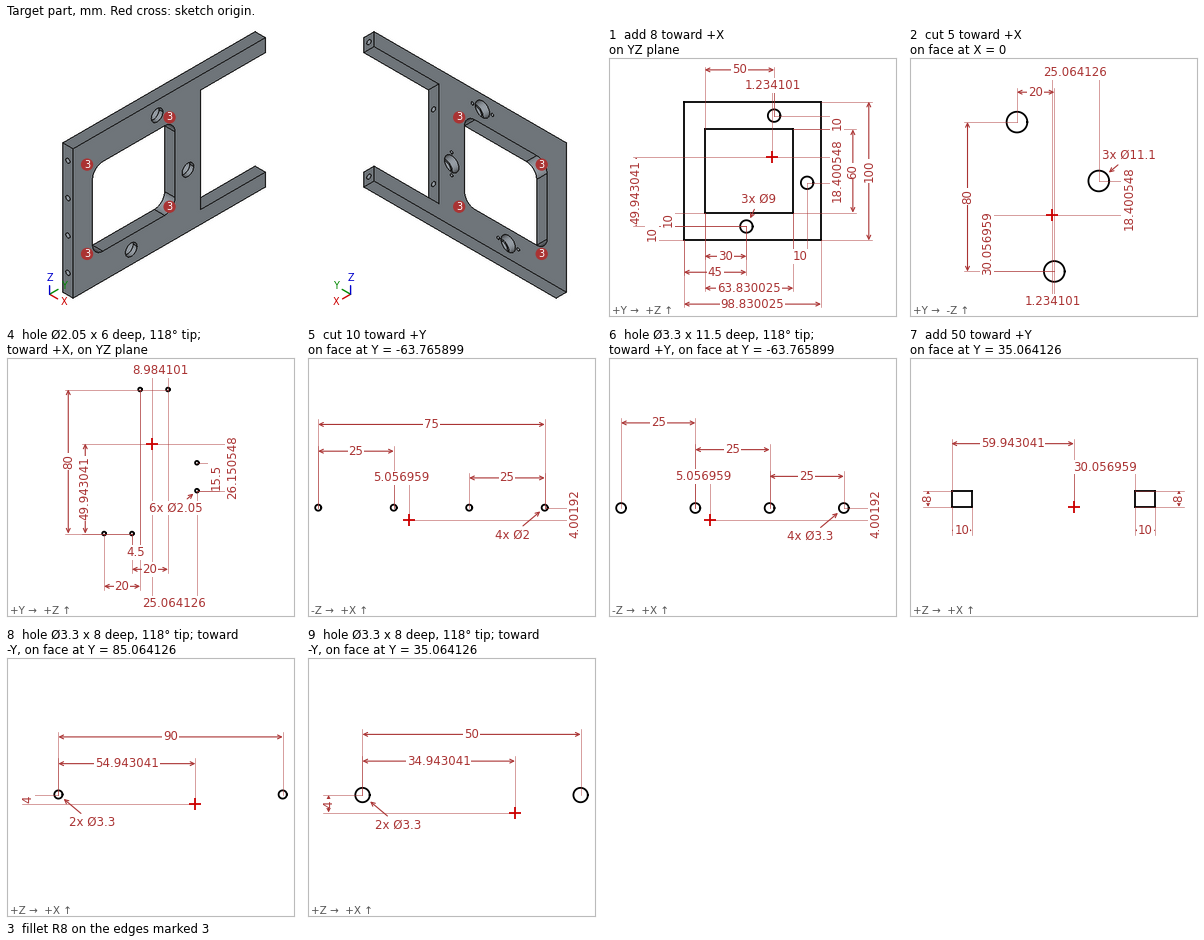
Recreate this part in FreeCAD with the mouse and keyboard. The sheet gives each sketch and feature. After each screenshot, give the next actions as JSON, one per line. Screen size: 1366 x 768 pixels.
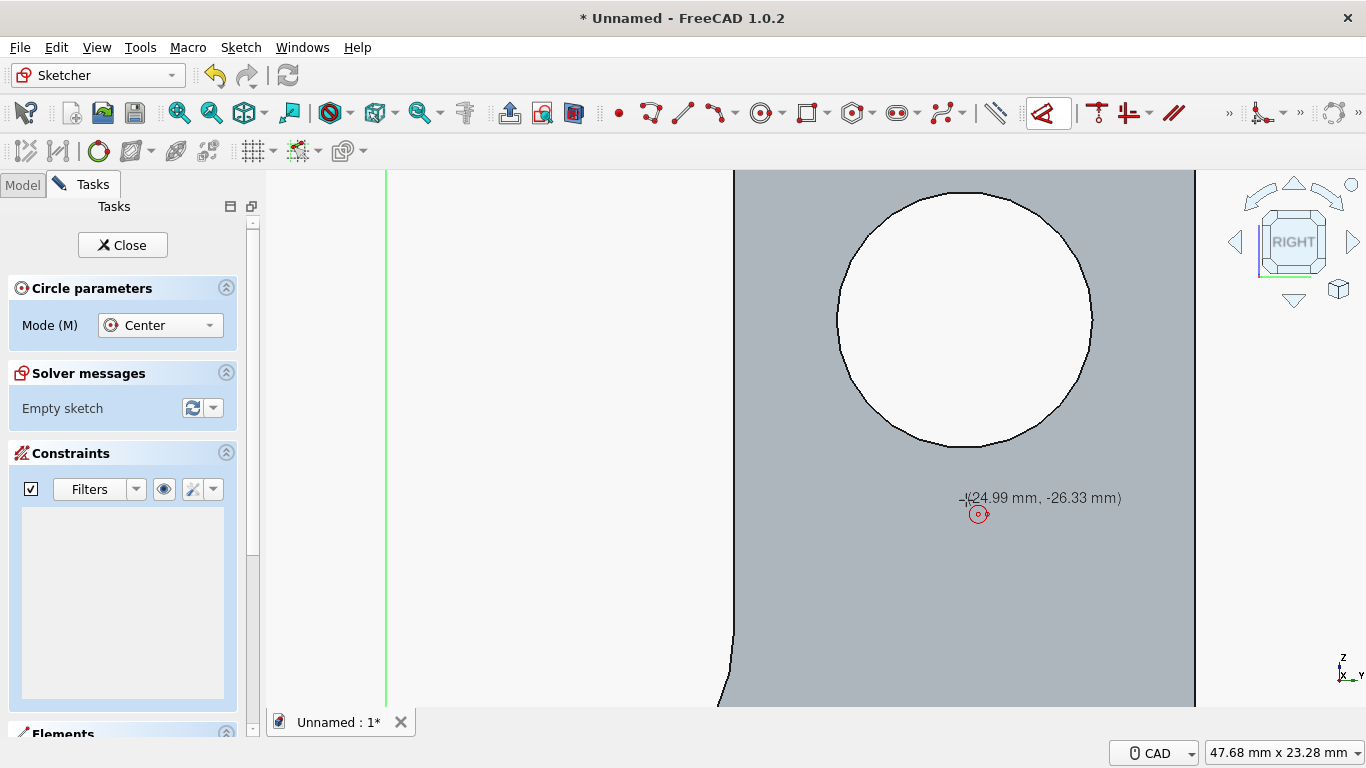
{"action": "scroll", "coordinate": [822, 501], "scroll_direction": "down", "scroll_amount": 9}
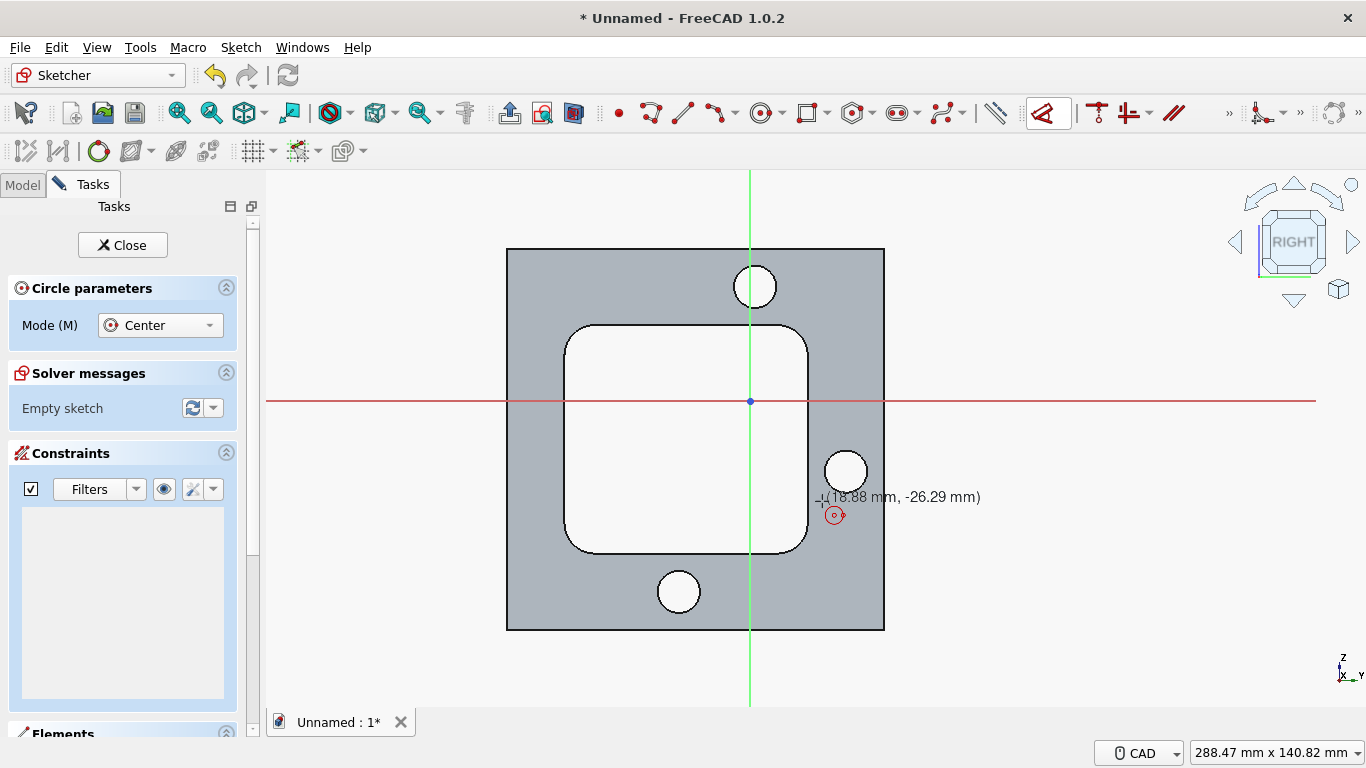
{"action": "left_click", "coordinate": [846, 501]}
{"action": "mouse_move", "coordinate": [849, 498]}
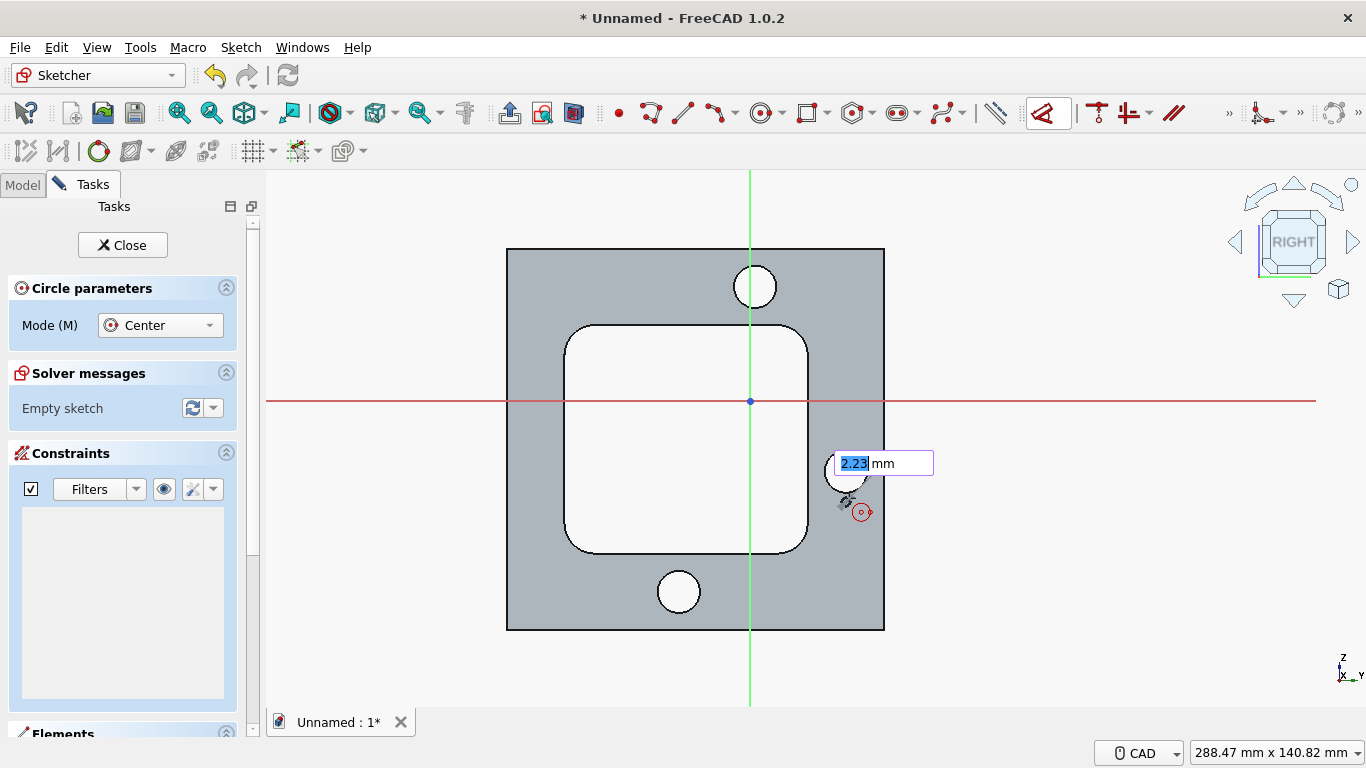
{"action": "type", "text": "2.05"}
{"action": "key", "text": "Return"}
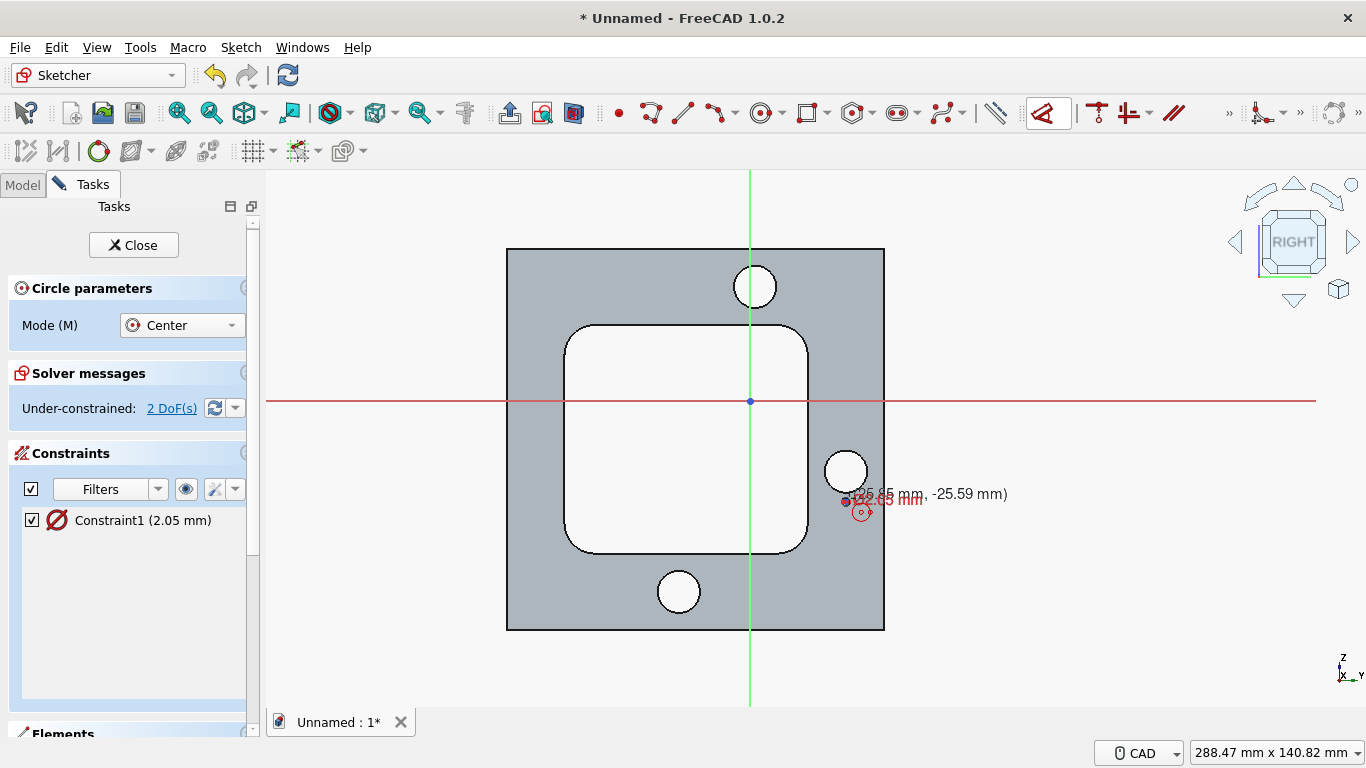
{"action": "scroll", "coordinate": [846, 442], "scroll_direction": "up", "scroll_amount": 9}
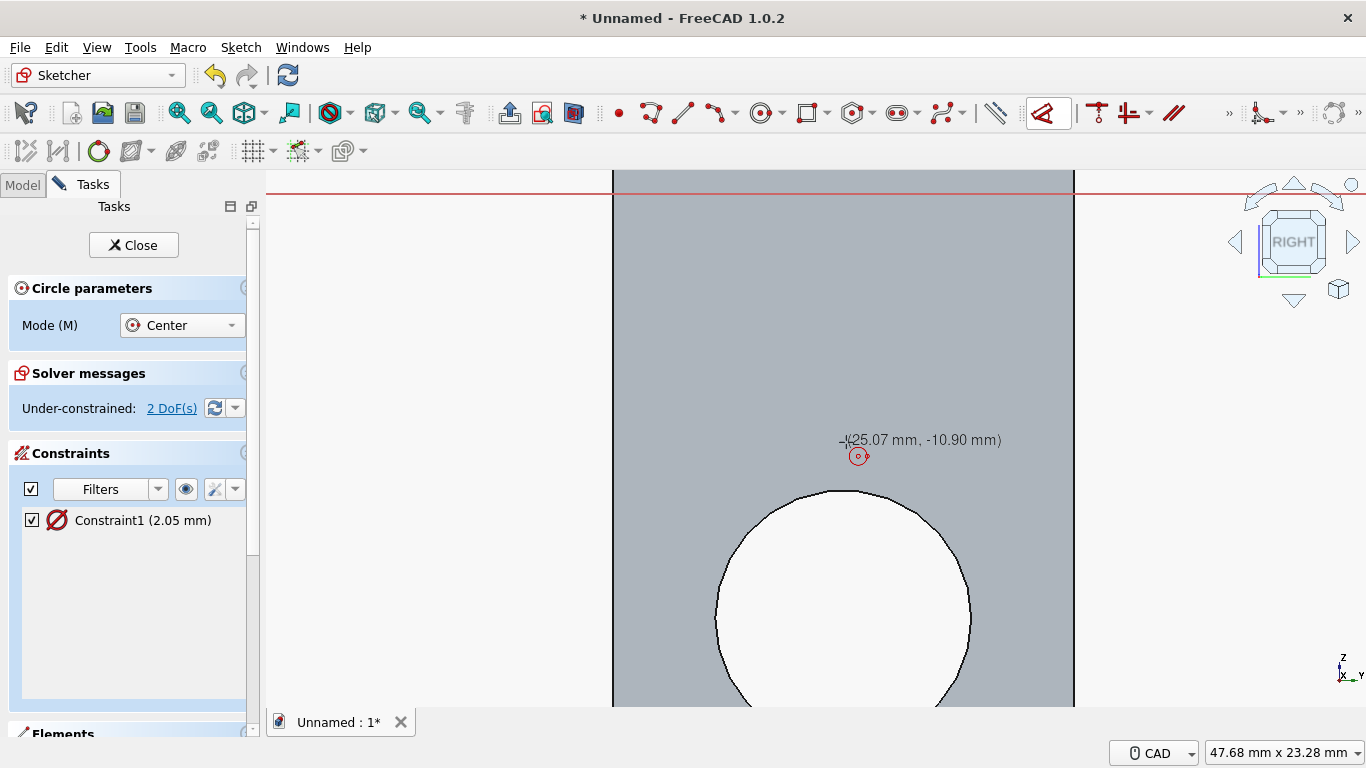
{"action": "scroll", "coordinate": [846, 442], "scroll_direction": "down", "scroll_amount": 9}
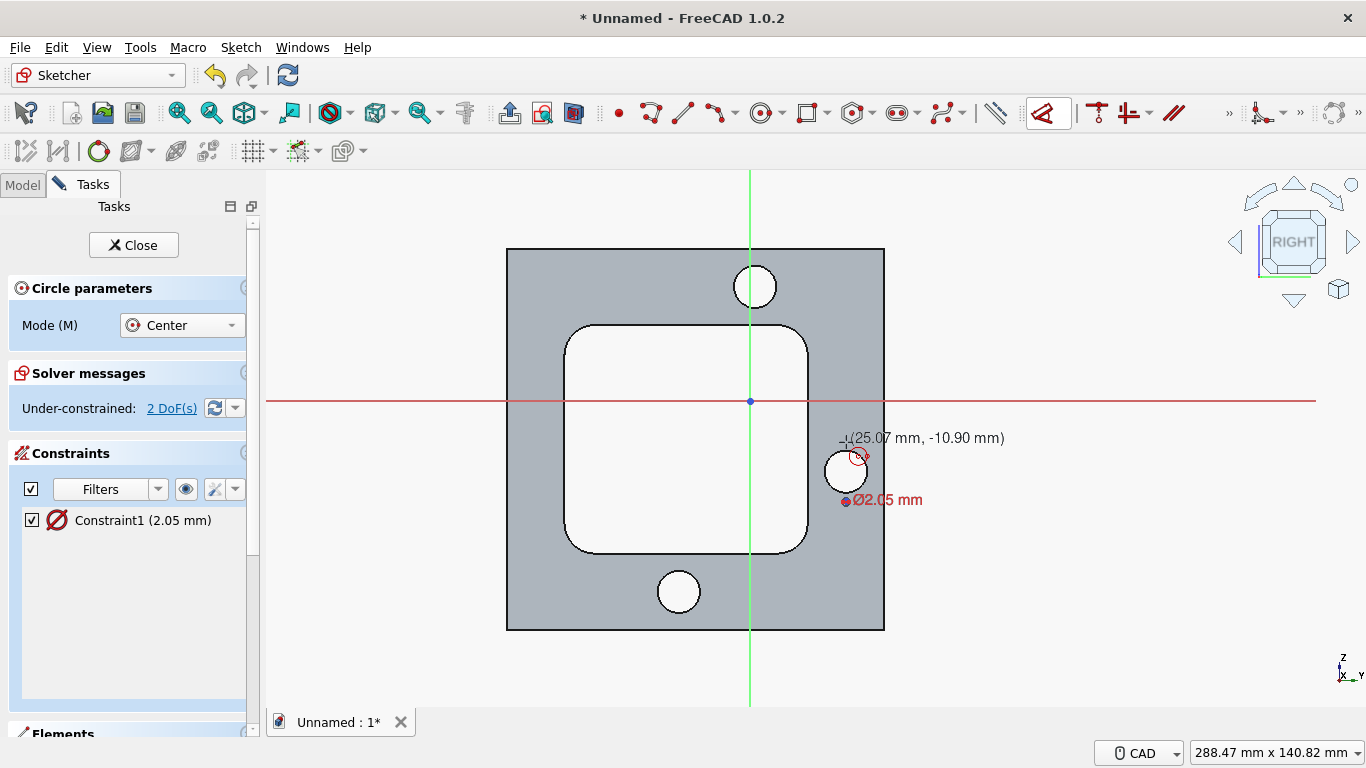
{"action": "left_click", "coordinate": [846, 442]}
{"action": "mouse_move", "coordinate": [849, 439]}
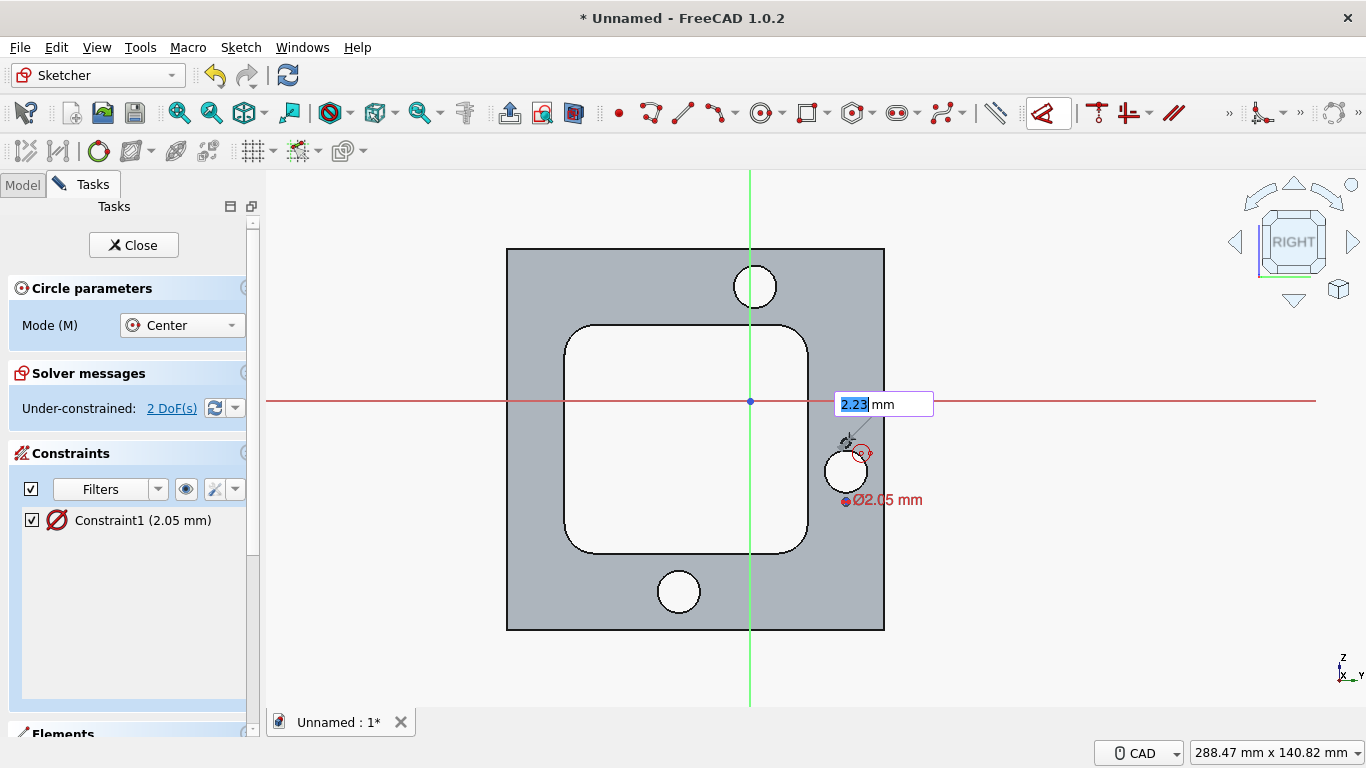
{"action": "type", "text": "2.05"}
{"action": "key", "text": "Return"}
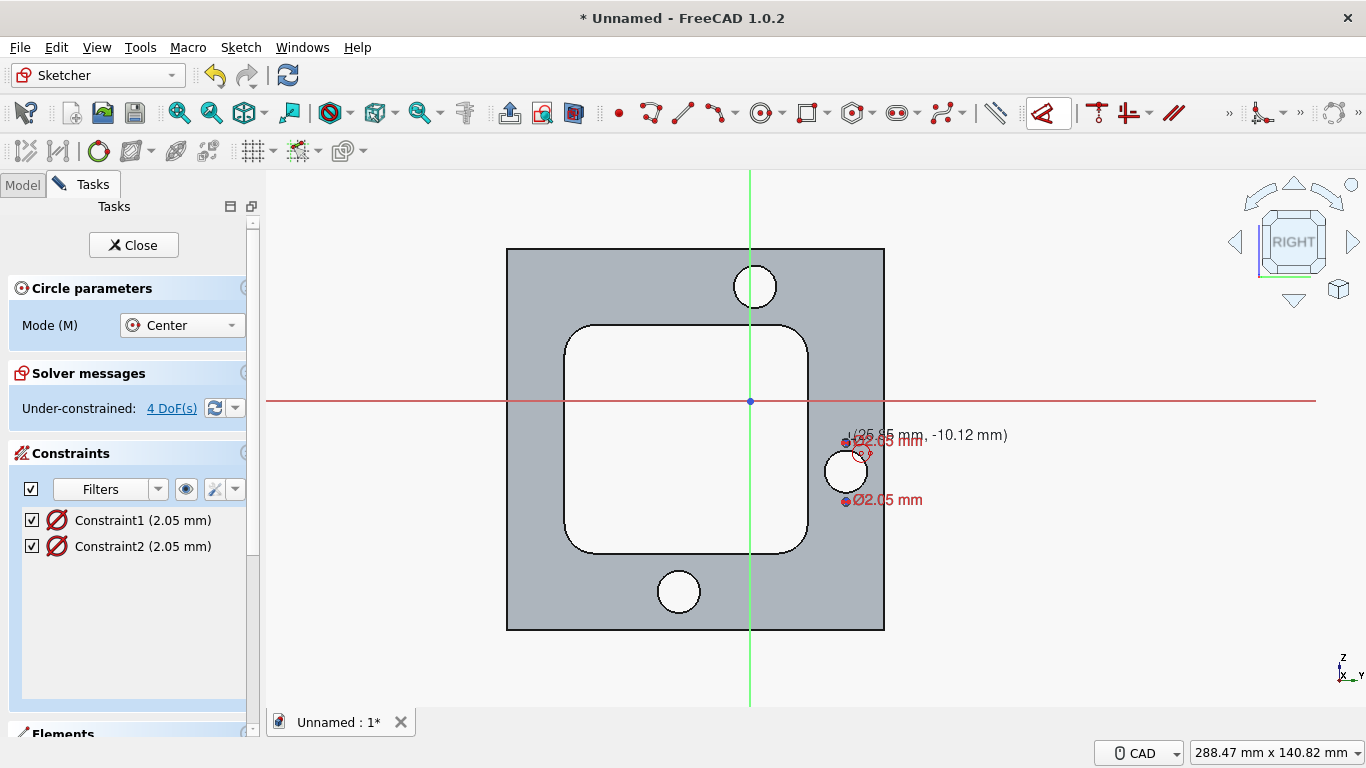
{"action": "scroll", "coordinate": [708, 592], "scroll_direction": "up", "scroll_amount": 9}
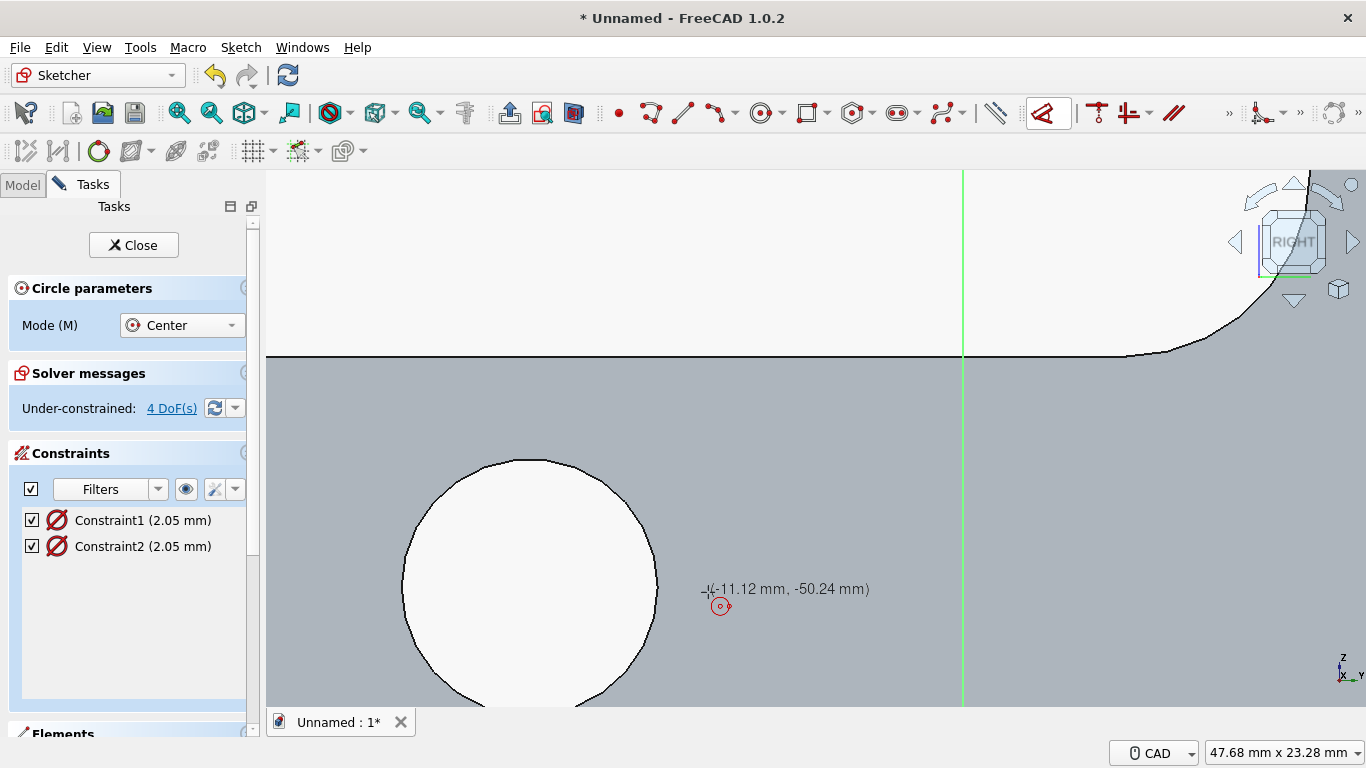
{"action": "scroll", "coordinate": [708, 592], "scroll_direction": "down", "scroll_amount": 9}